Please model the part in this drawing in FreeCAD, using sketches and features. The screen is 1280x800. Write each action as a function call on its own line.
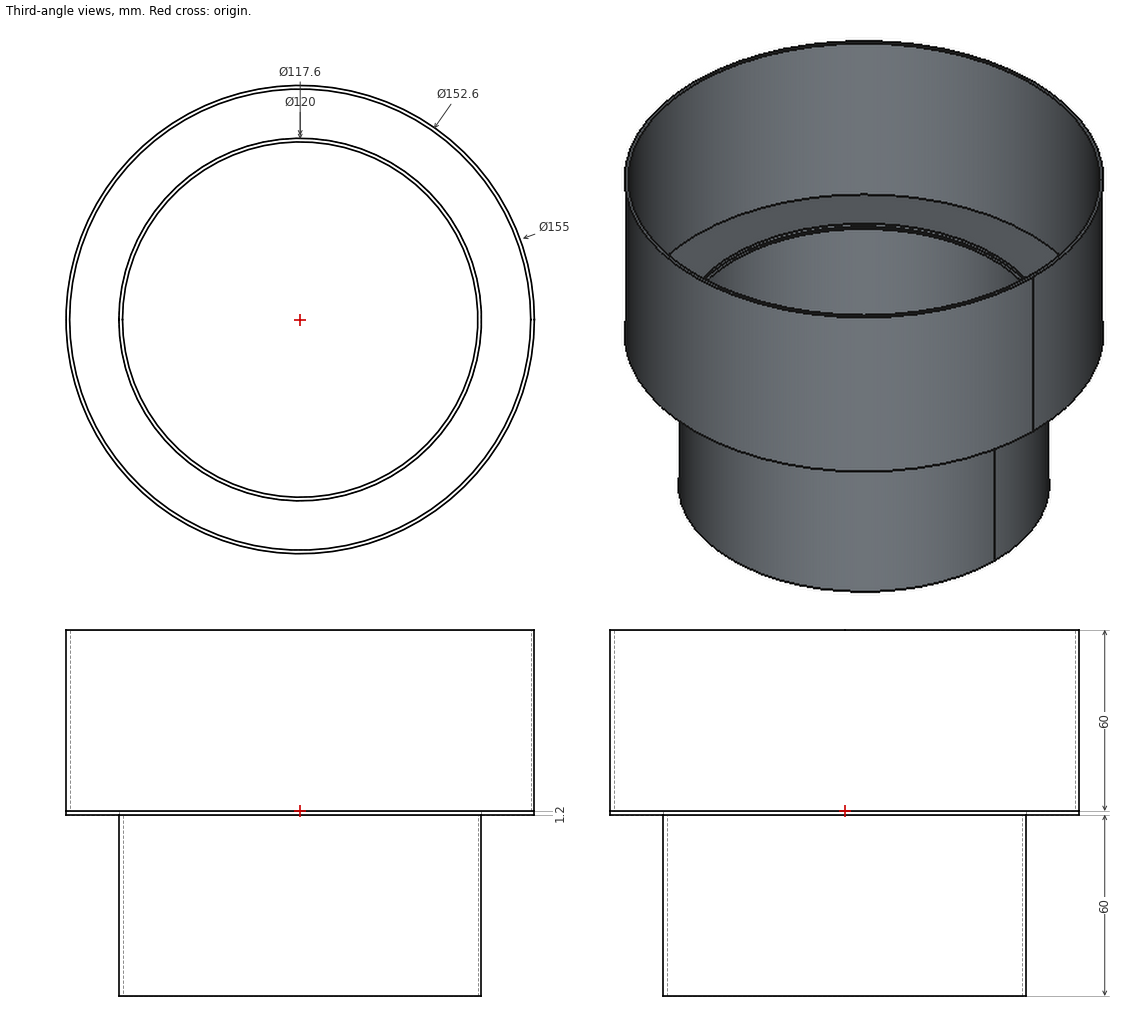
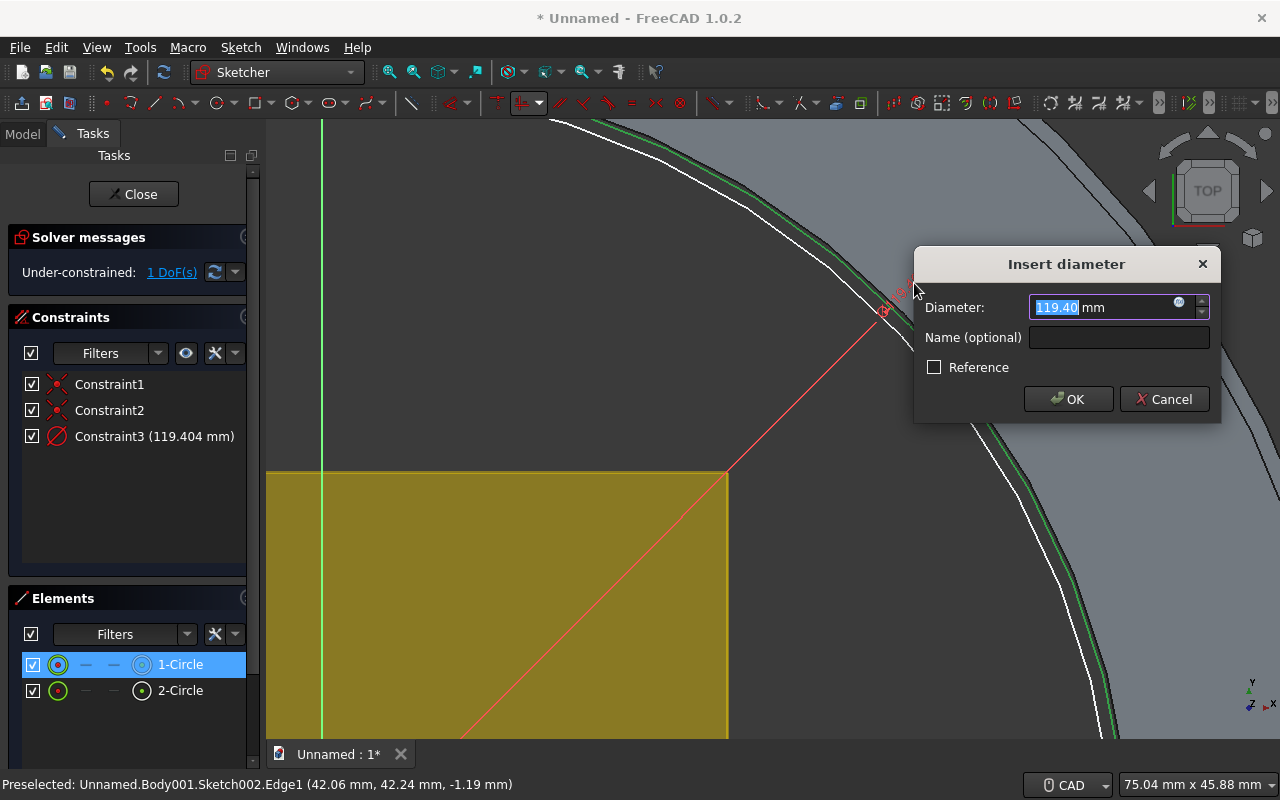
text(120)
key(Return)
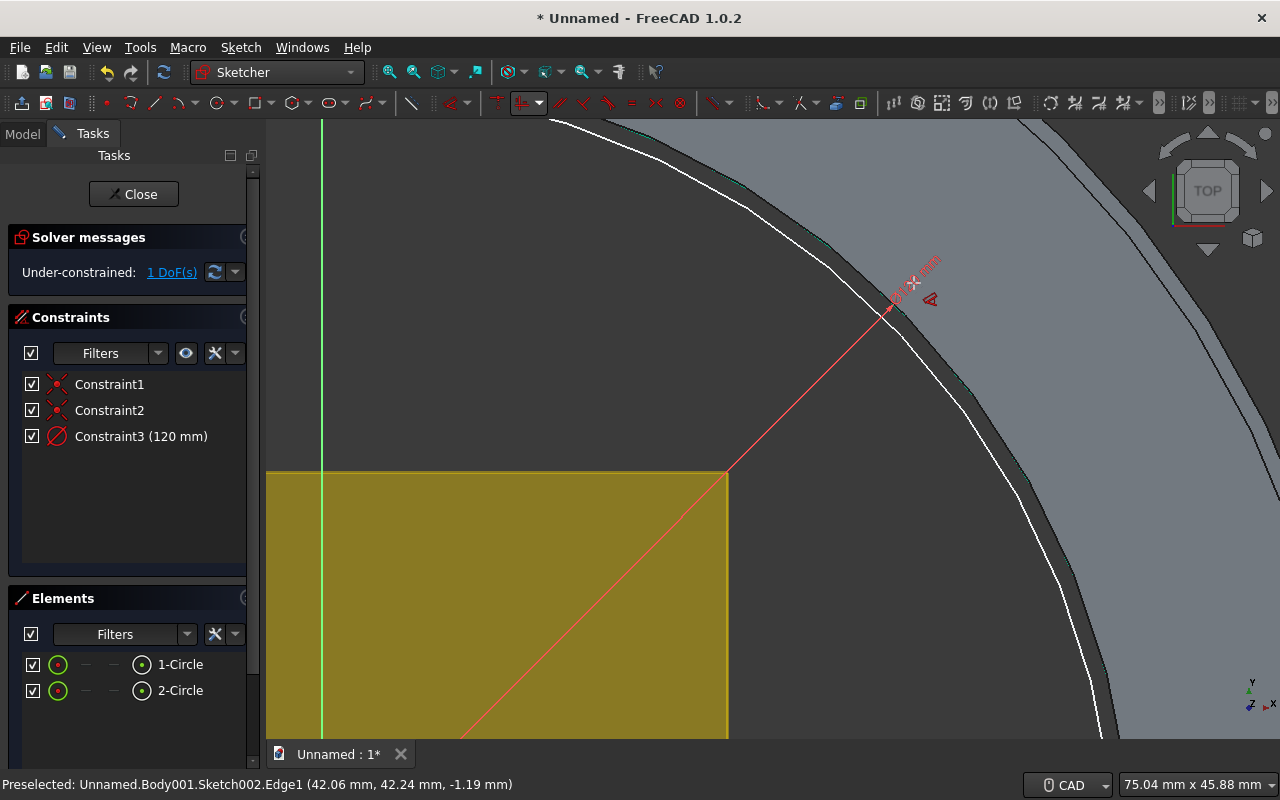
click(882, 316)
click(1114, 644)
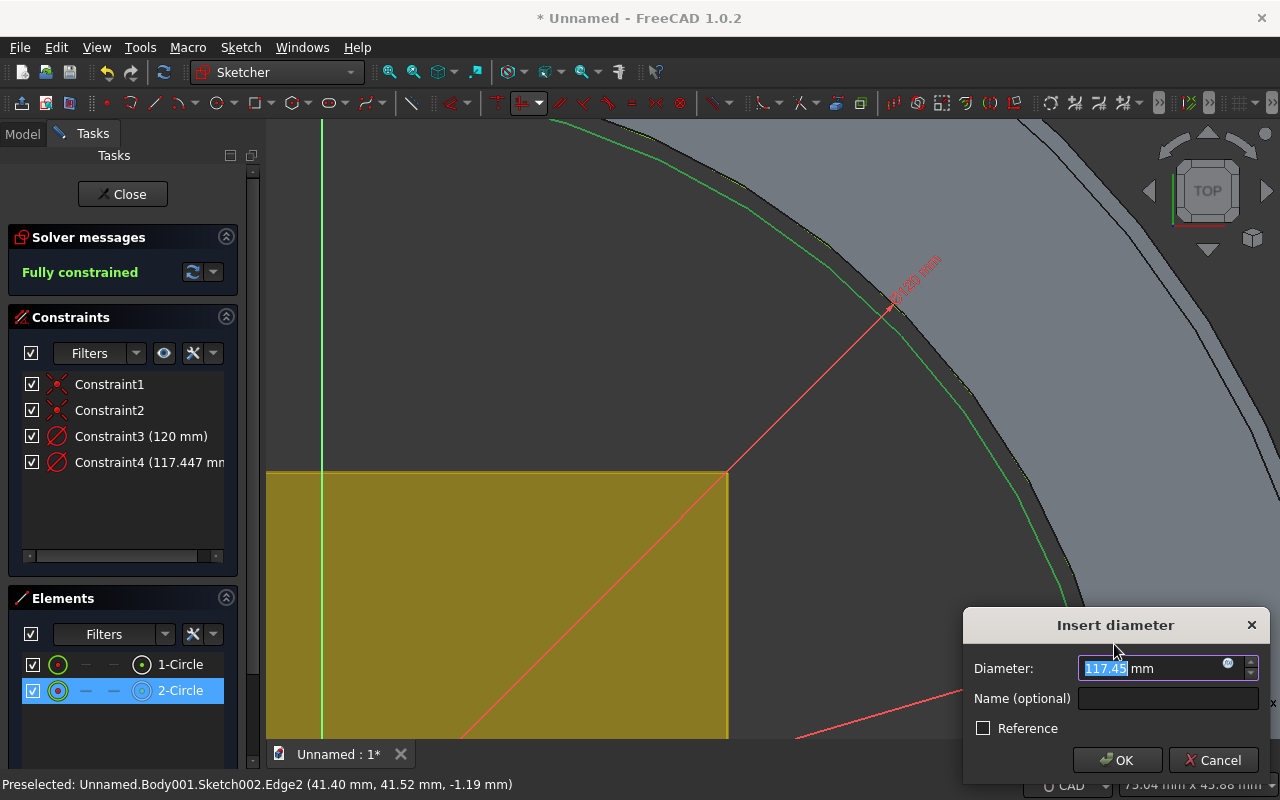
text(117.6)
key(Return)
key(Escape)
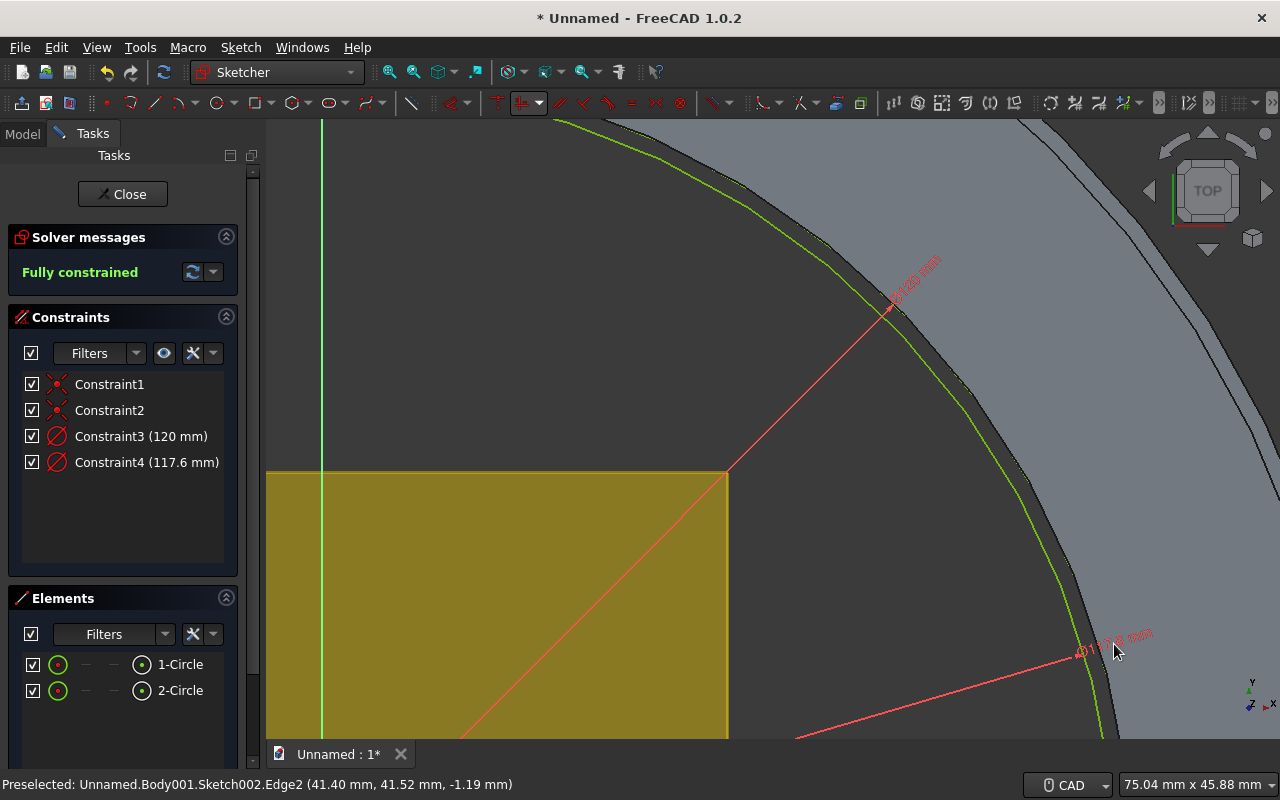
click(123, 194)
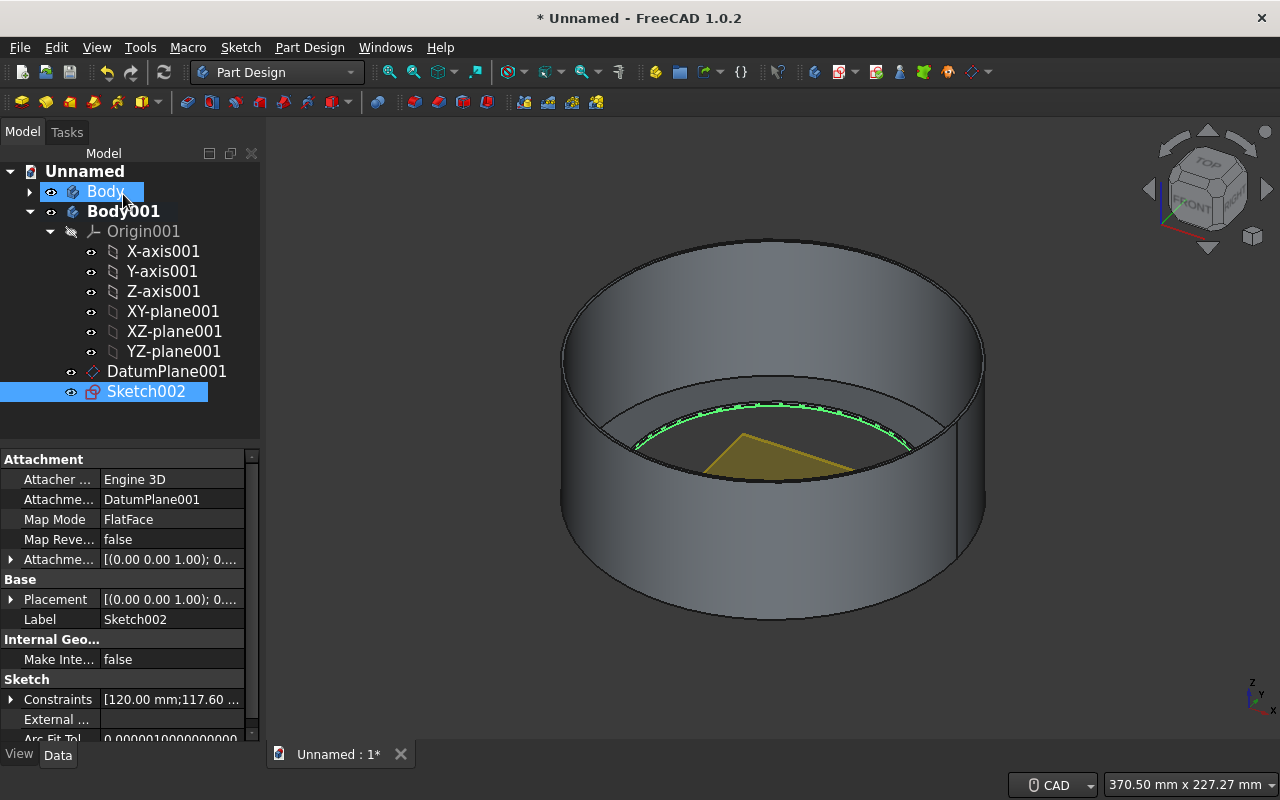
click(22, 102)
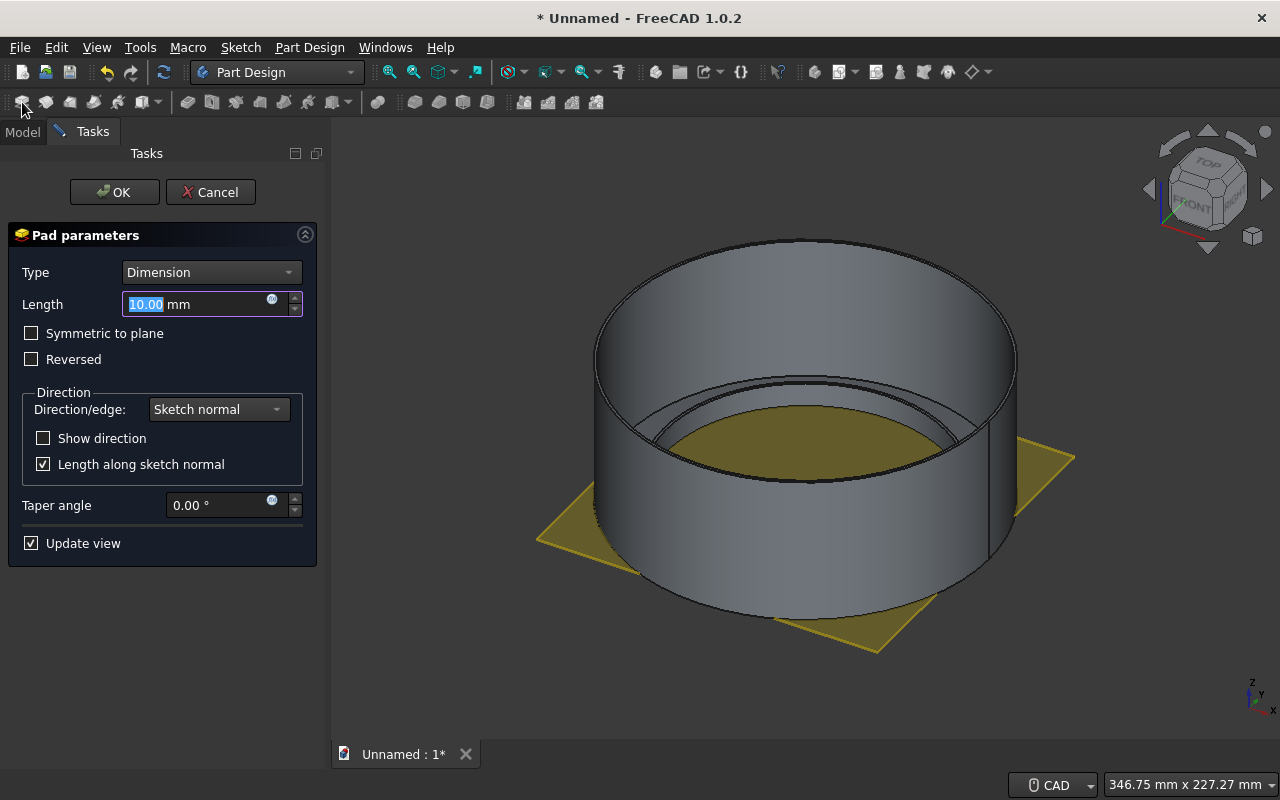
text(60)
key(Tab)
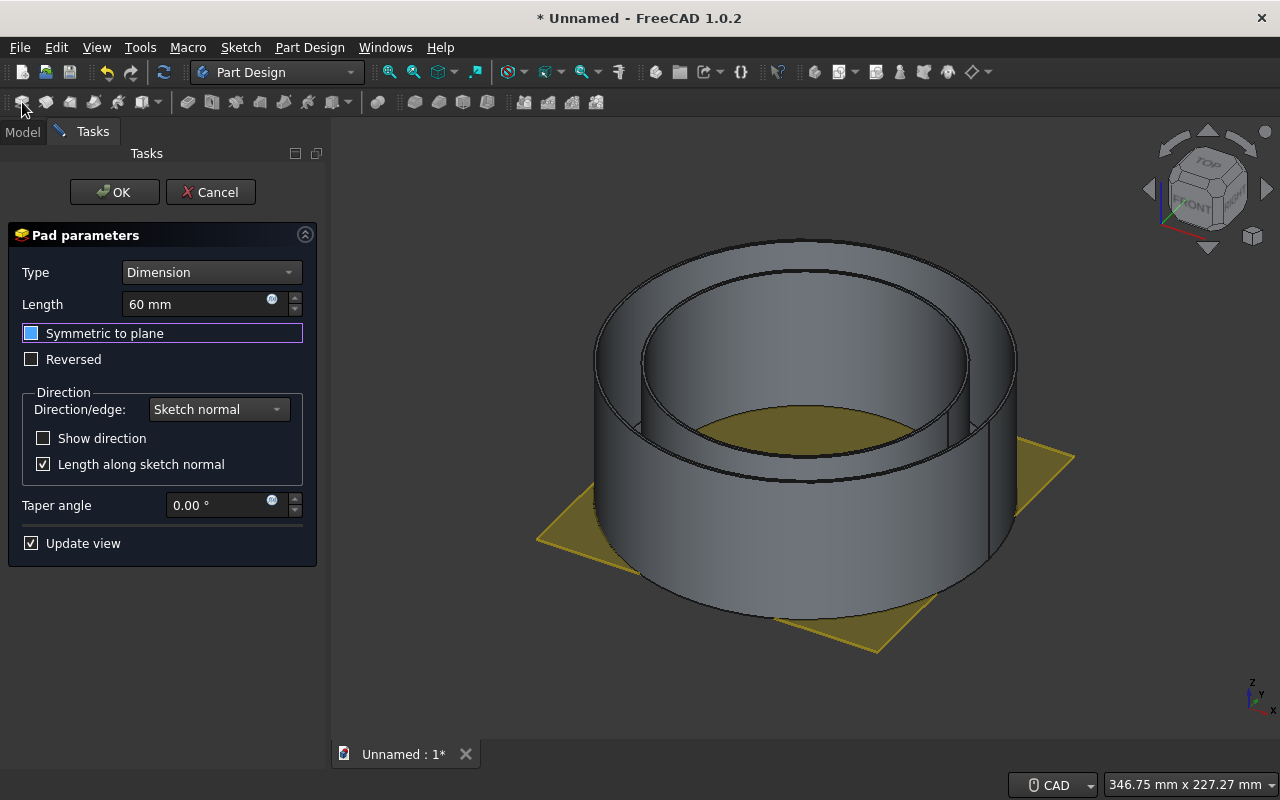
click(30, 359)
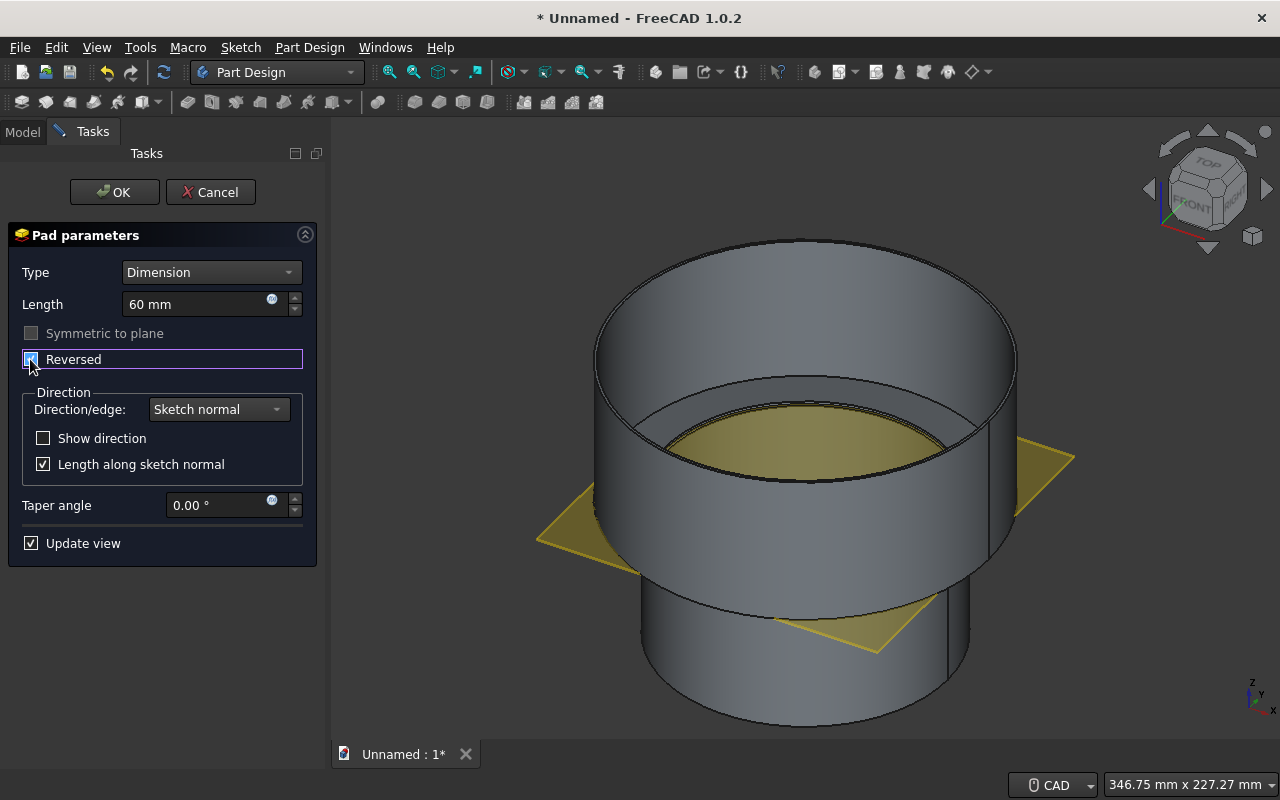
click(115, 192)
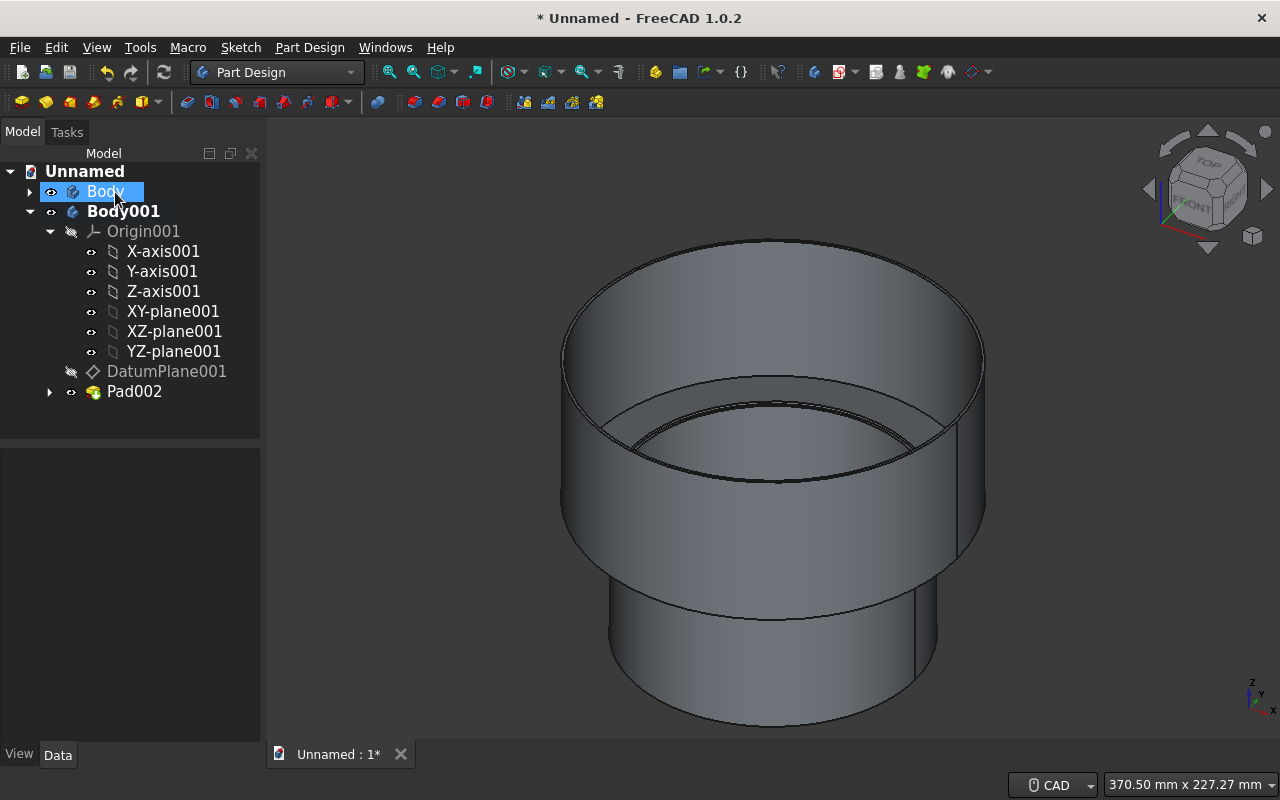
key(0)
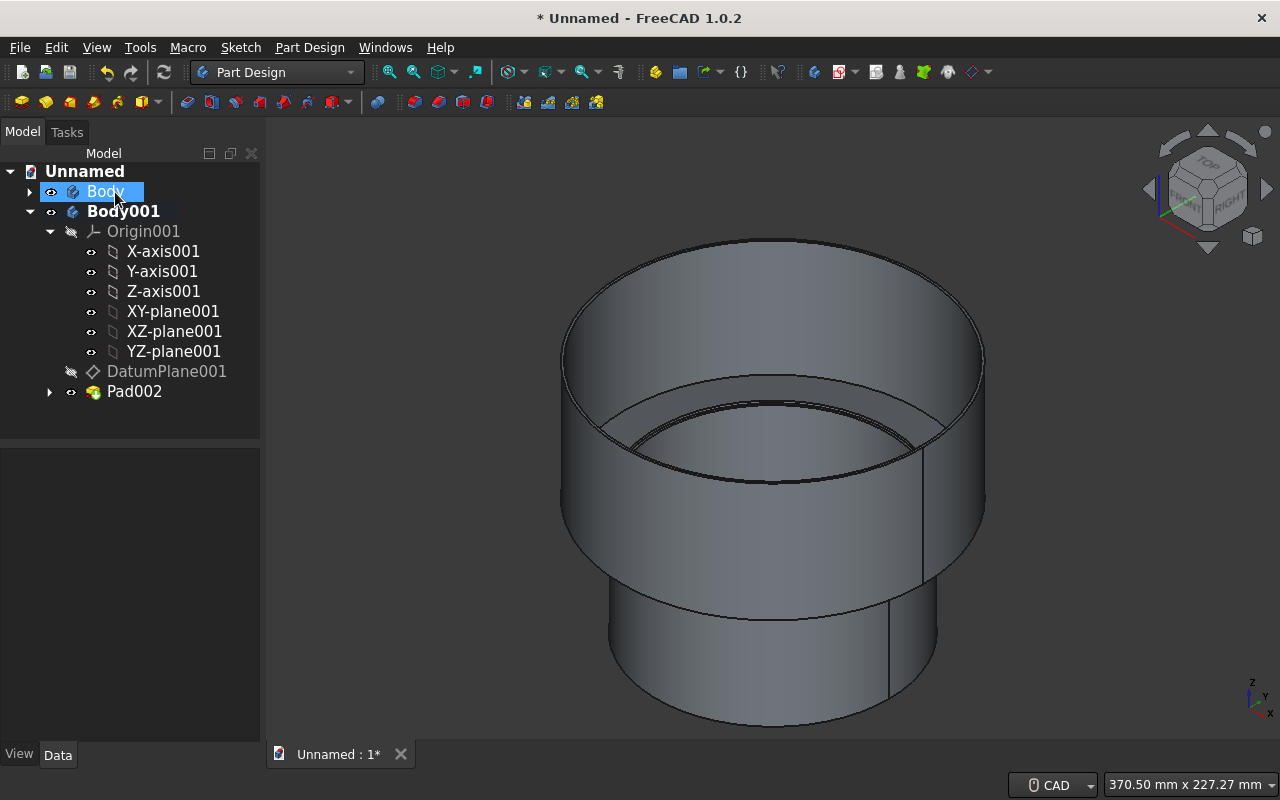
click(390, 72)